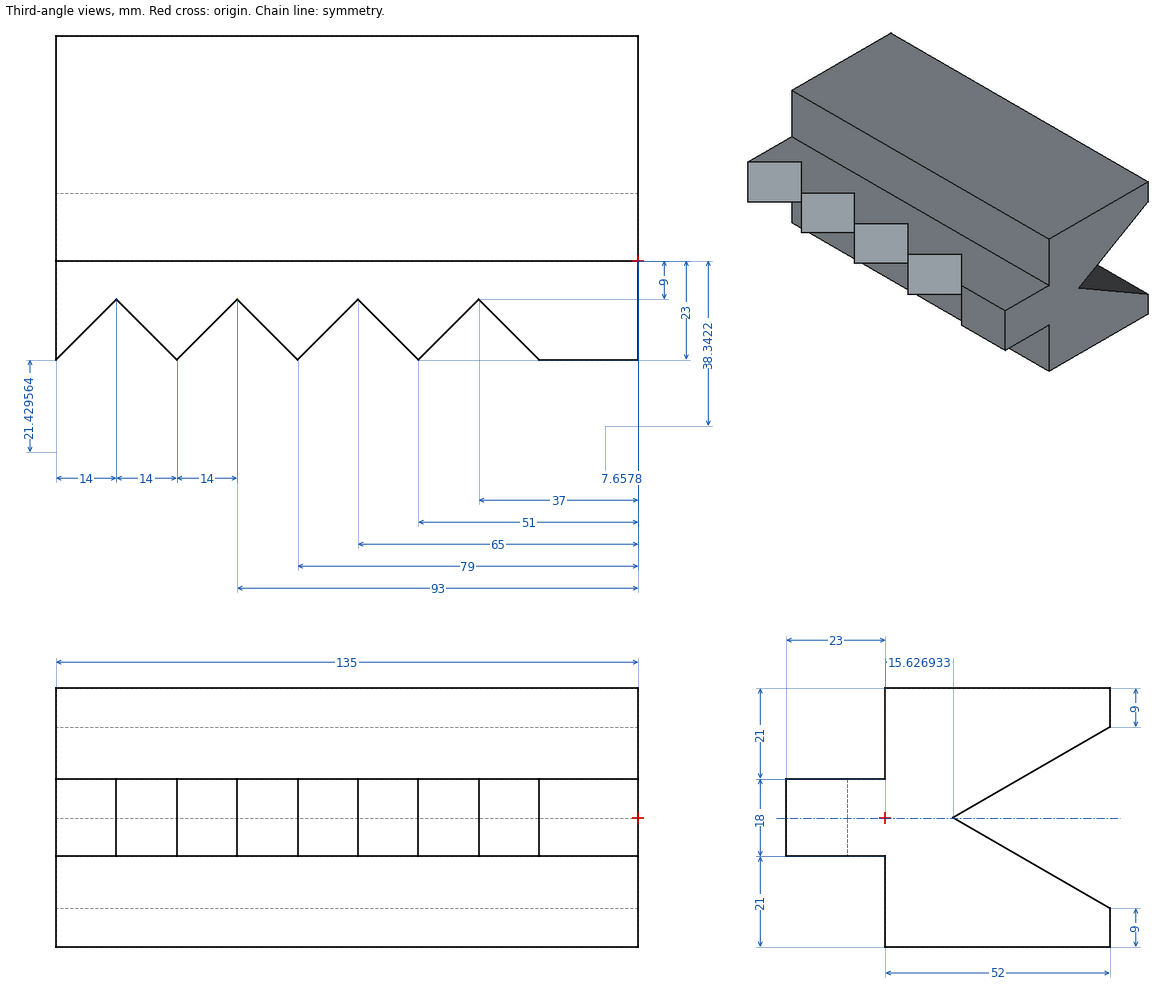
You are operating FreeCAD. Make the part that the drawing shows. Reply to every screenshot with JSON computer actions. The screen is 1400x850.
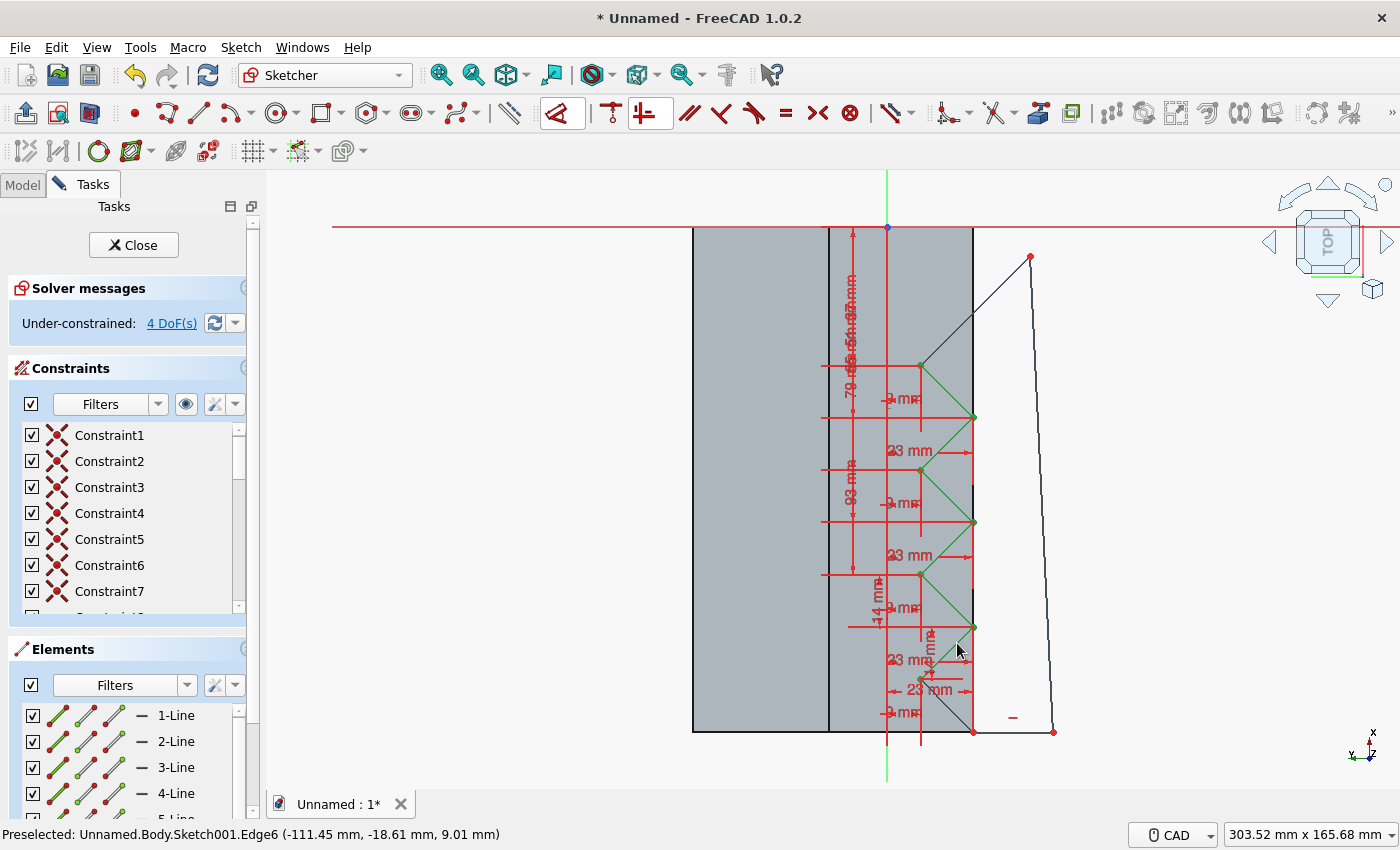
{"action": "left_click", "coordinate": [957, 717]}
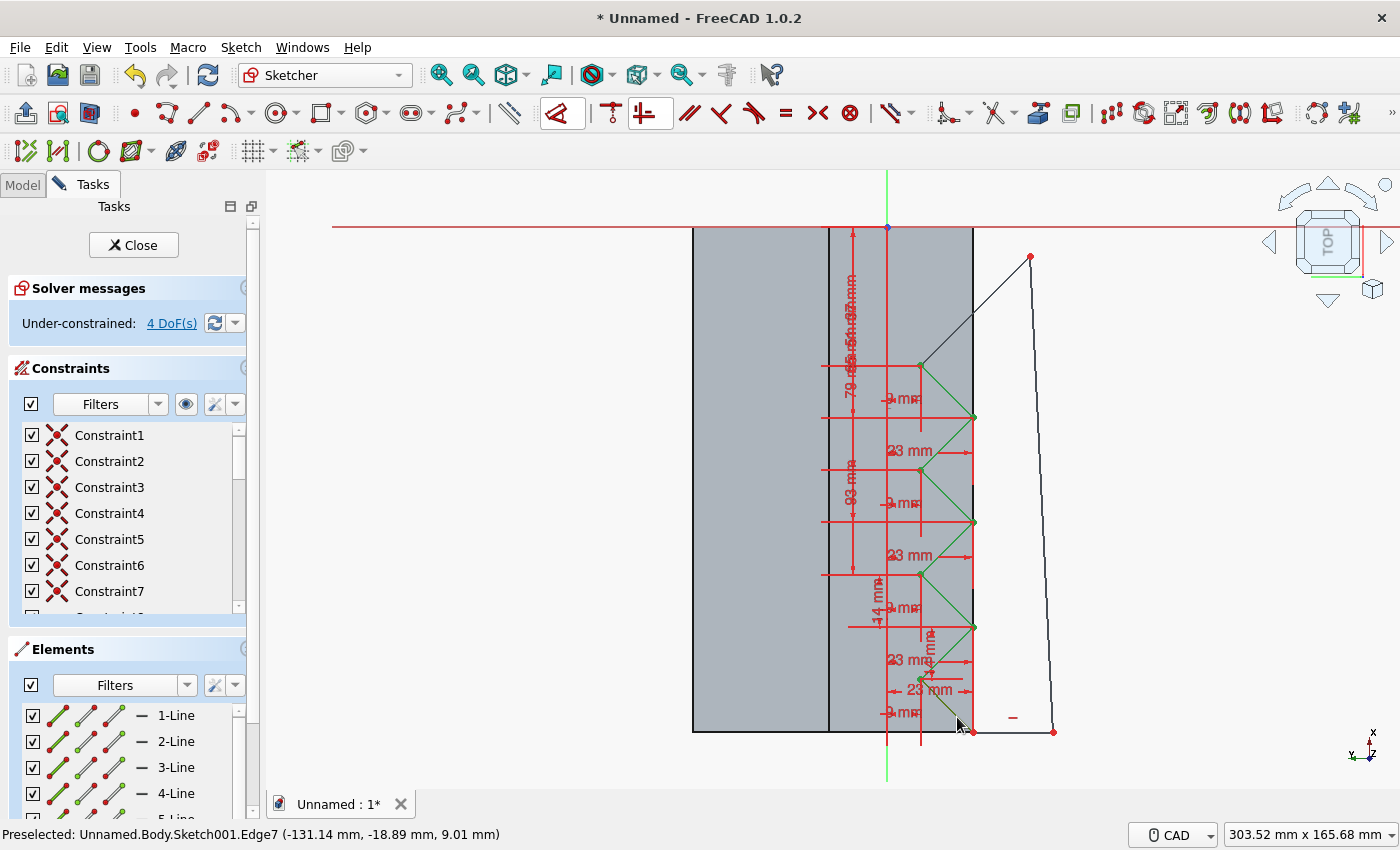
{"action": "left_click", "coordinate": [580, 114]}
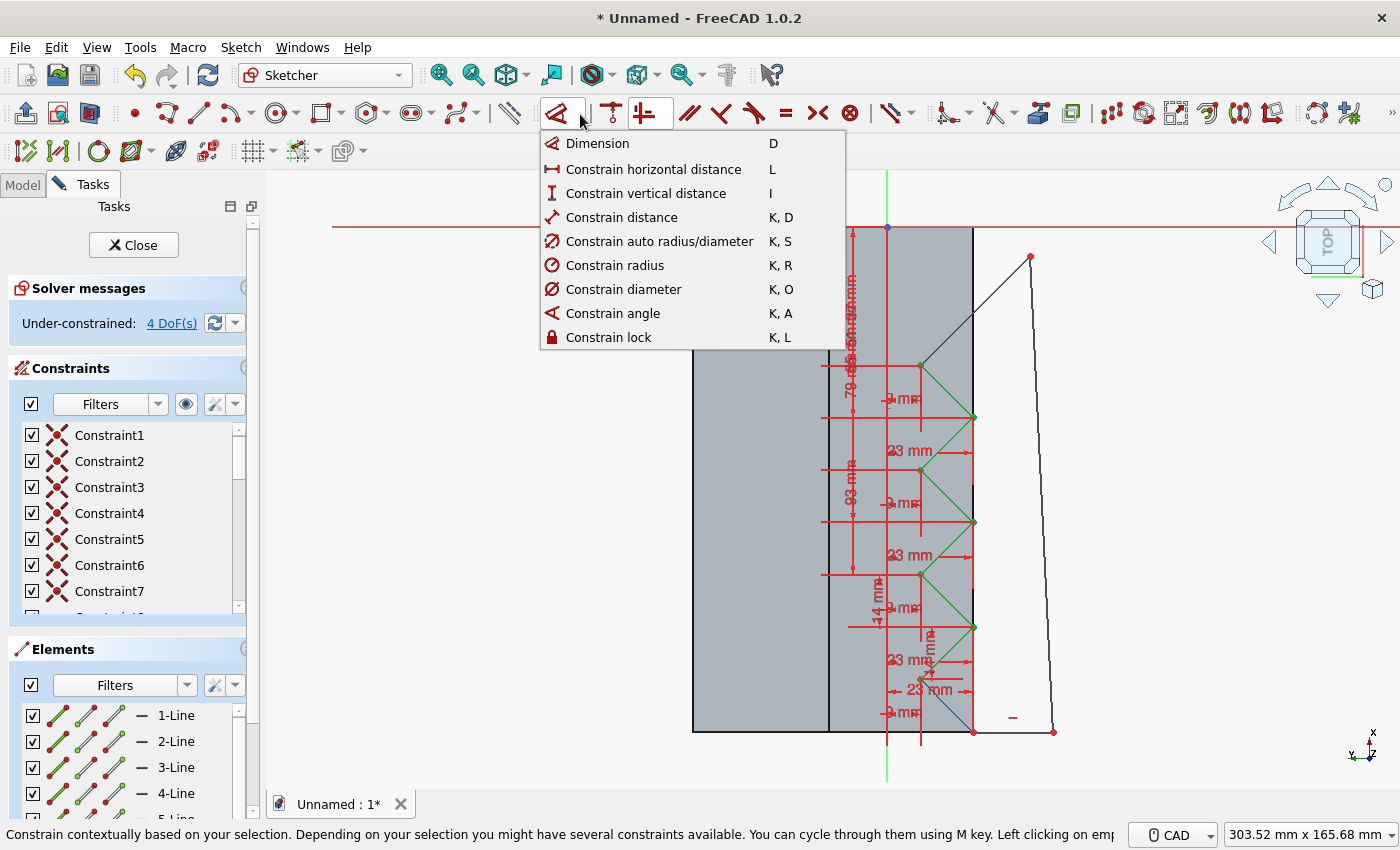
{"action": "left_click", "coordinate": [693, 193]}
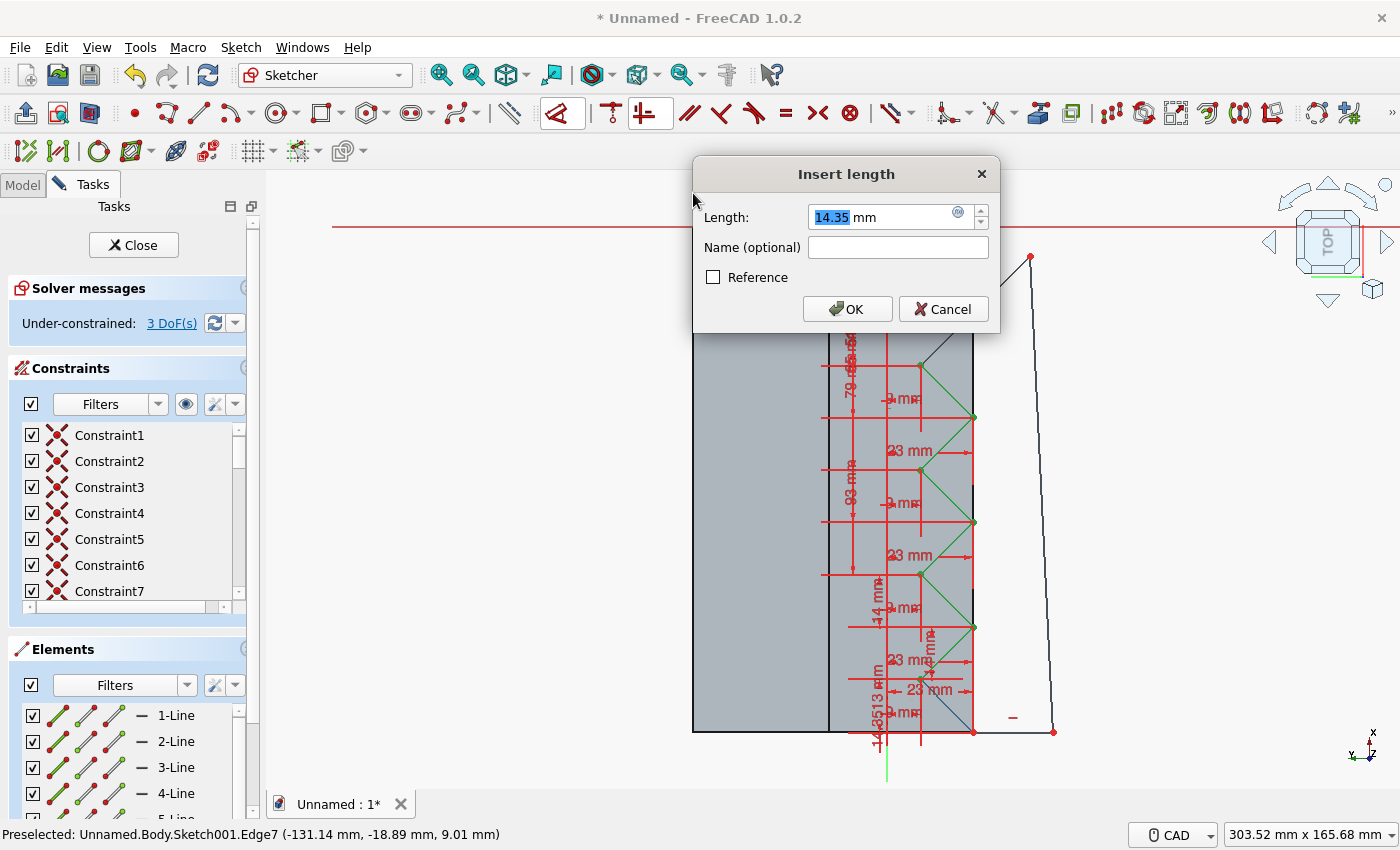
{"action": "type", "text": "14"}
{"action": "key", "text": "Return"}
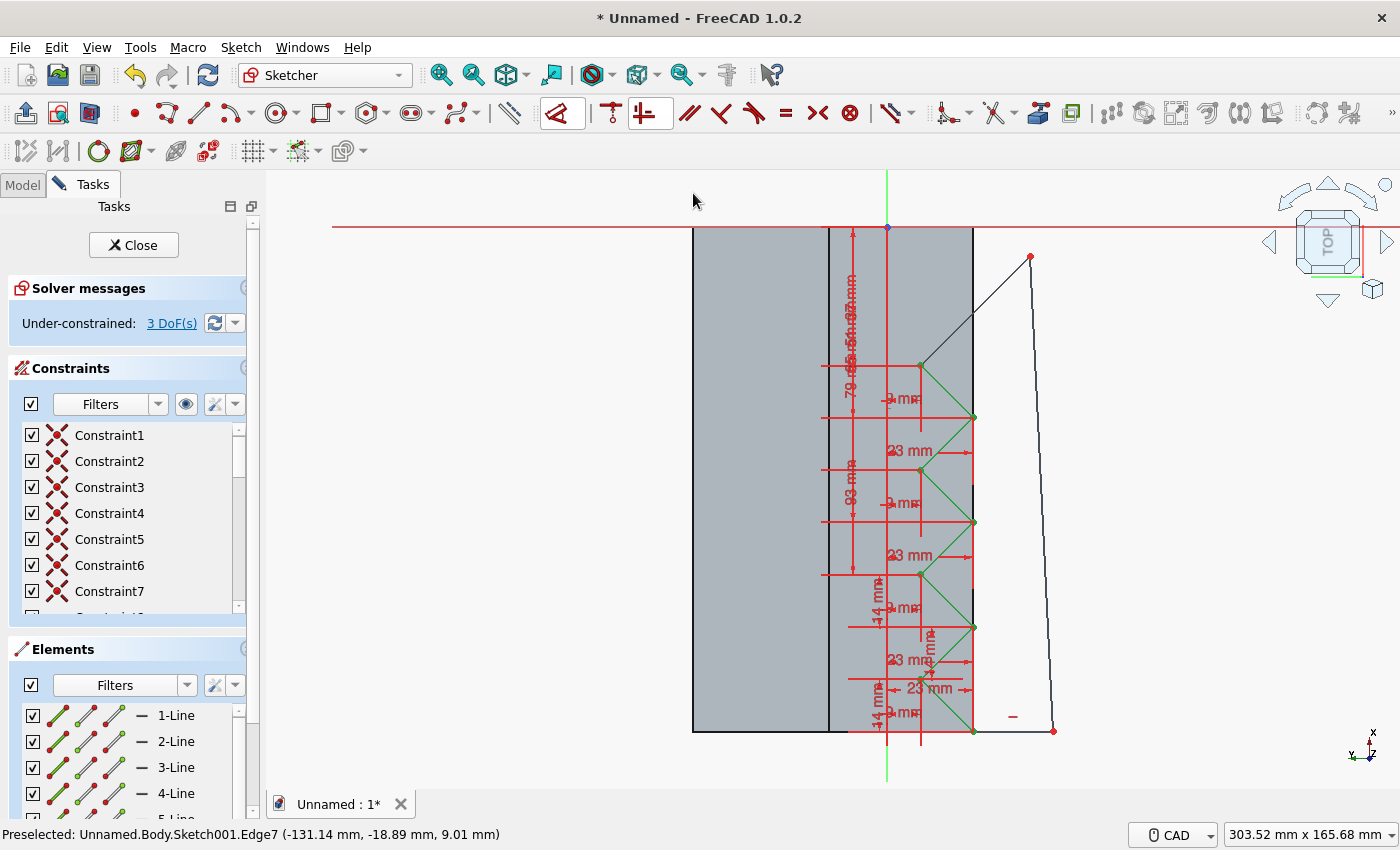
{"action": "scroll", "coordinate": [1030, 257], "scroll_direction": "up", "scroll_amount": 2}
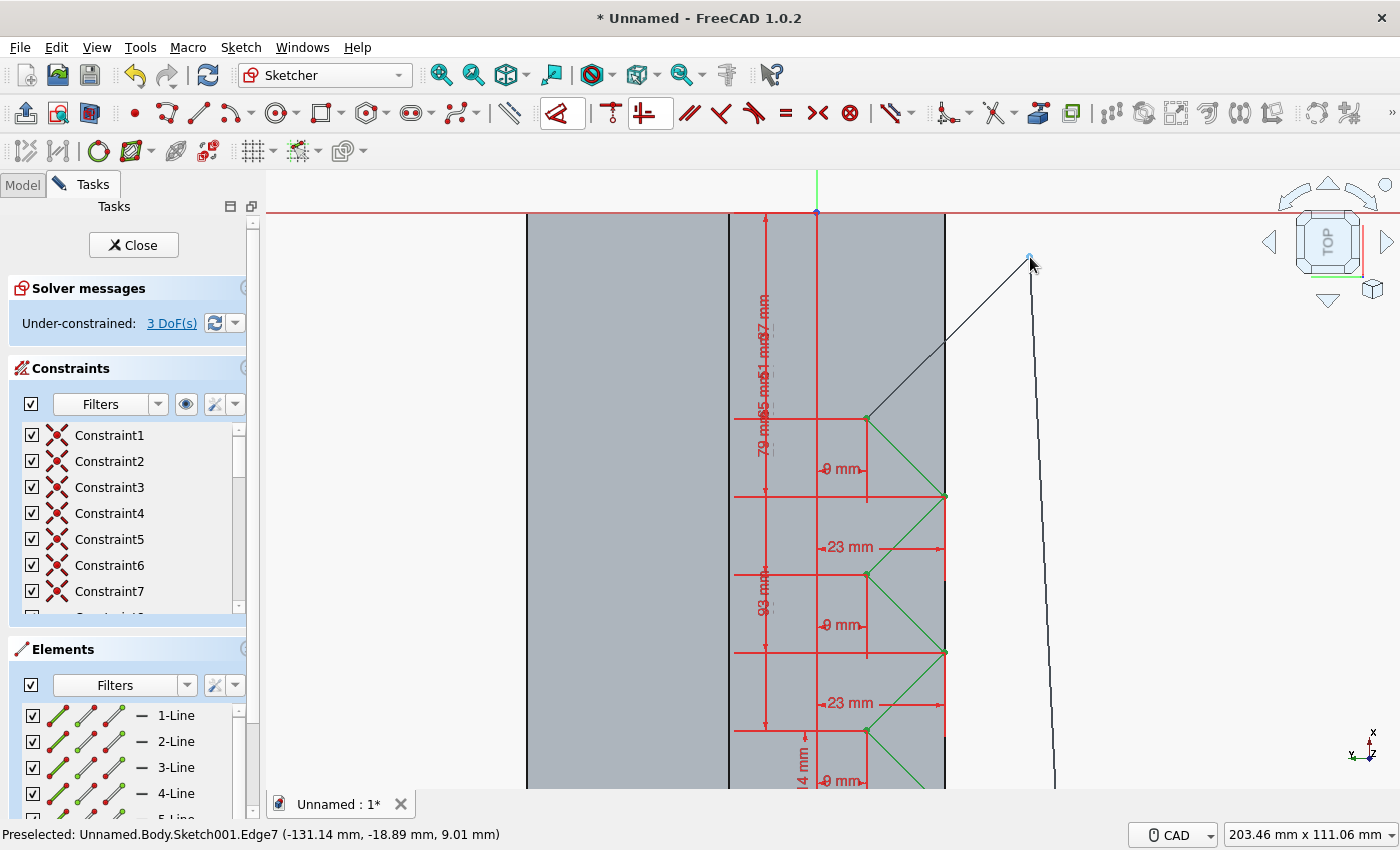
{"action": "left_click", "coordinate": [1030, 257]}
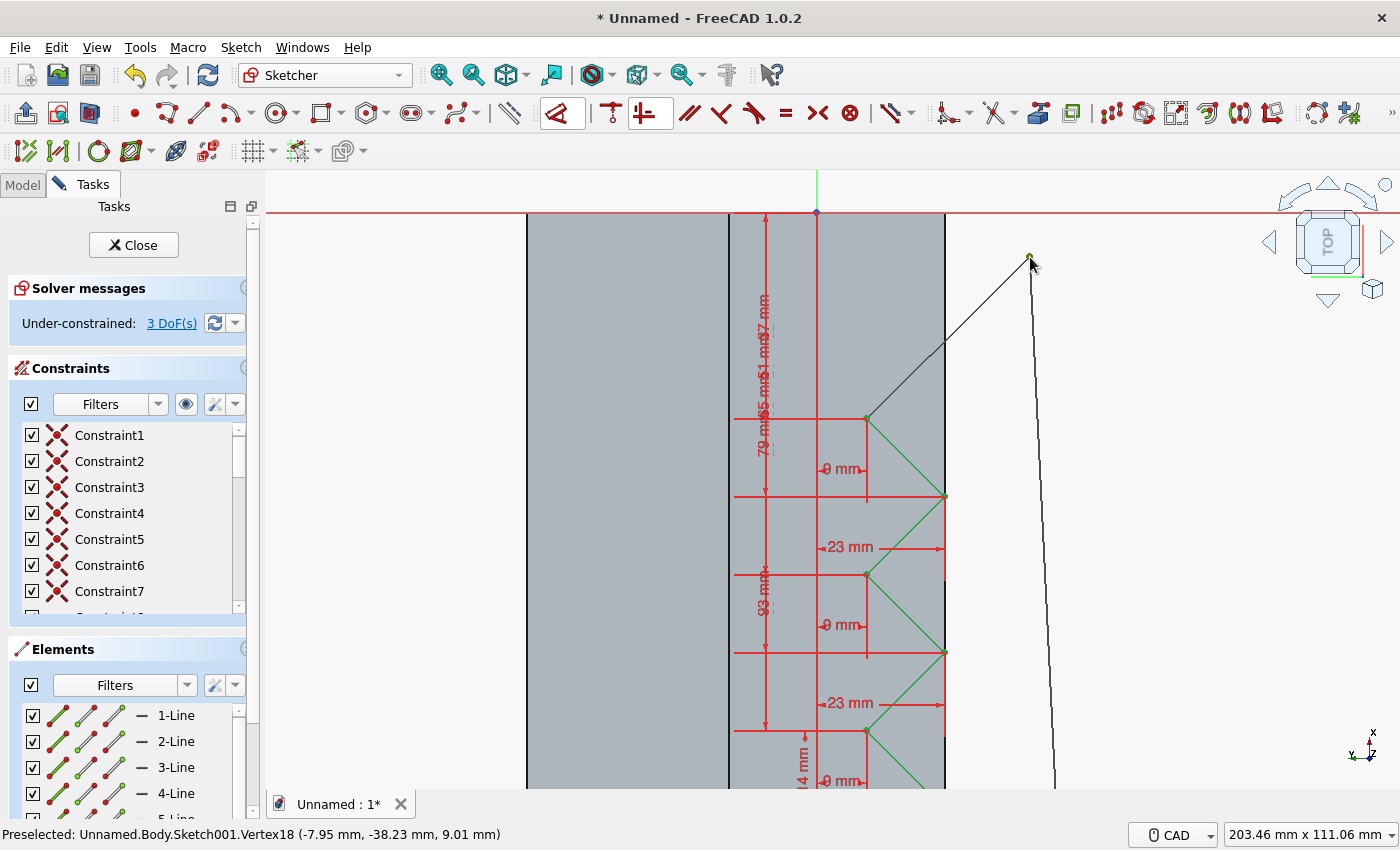
{"action": "left_click", "coordinate": [580, 114]}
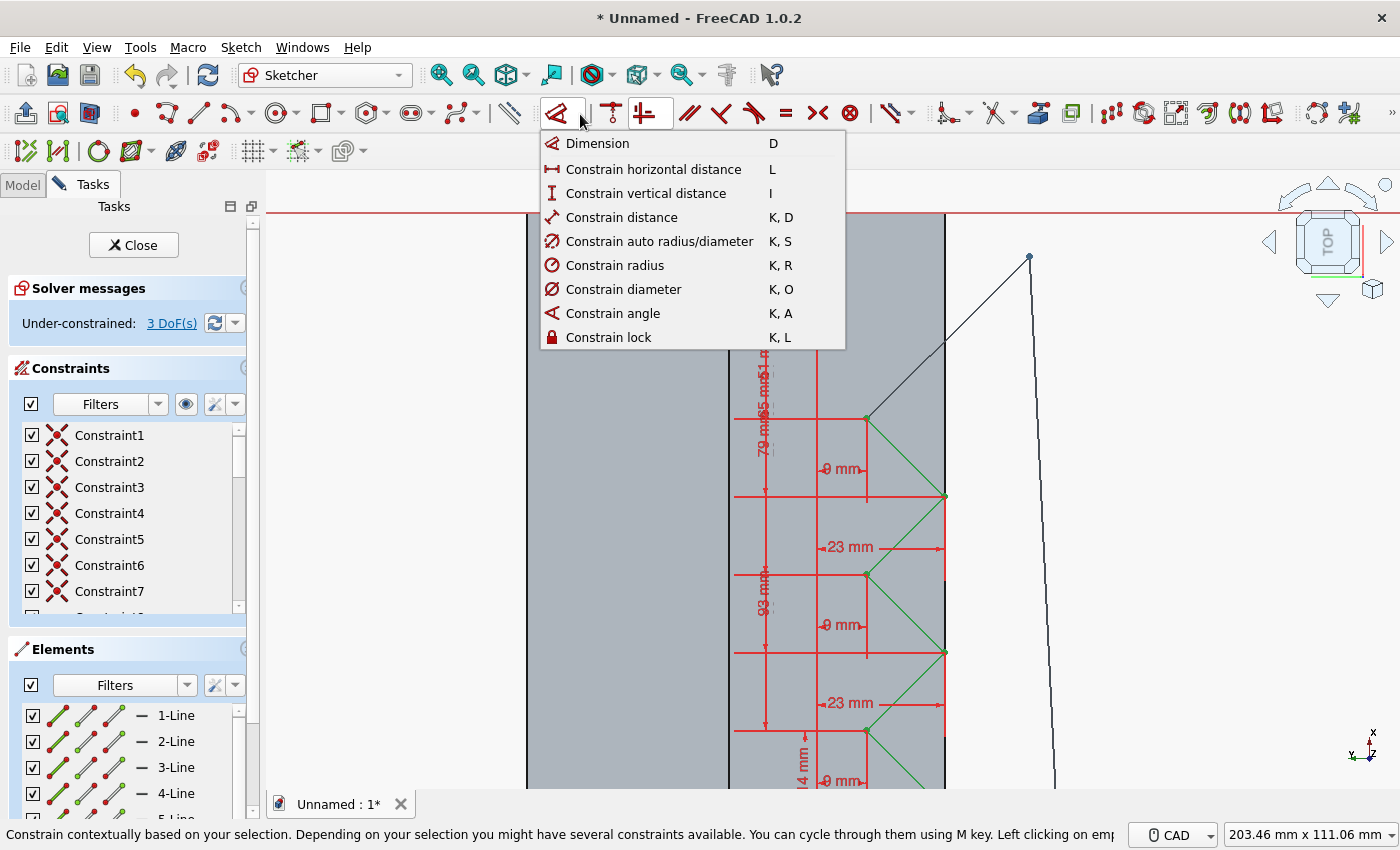
{"action": "left_click", "coordinate": [693, 193]}